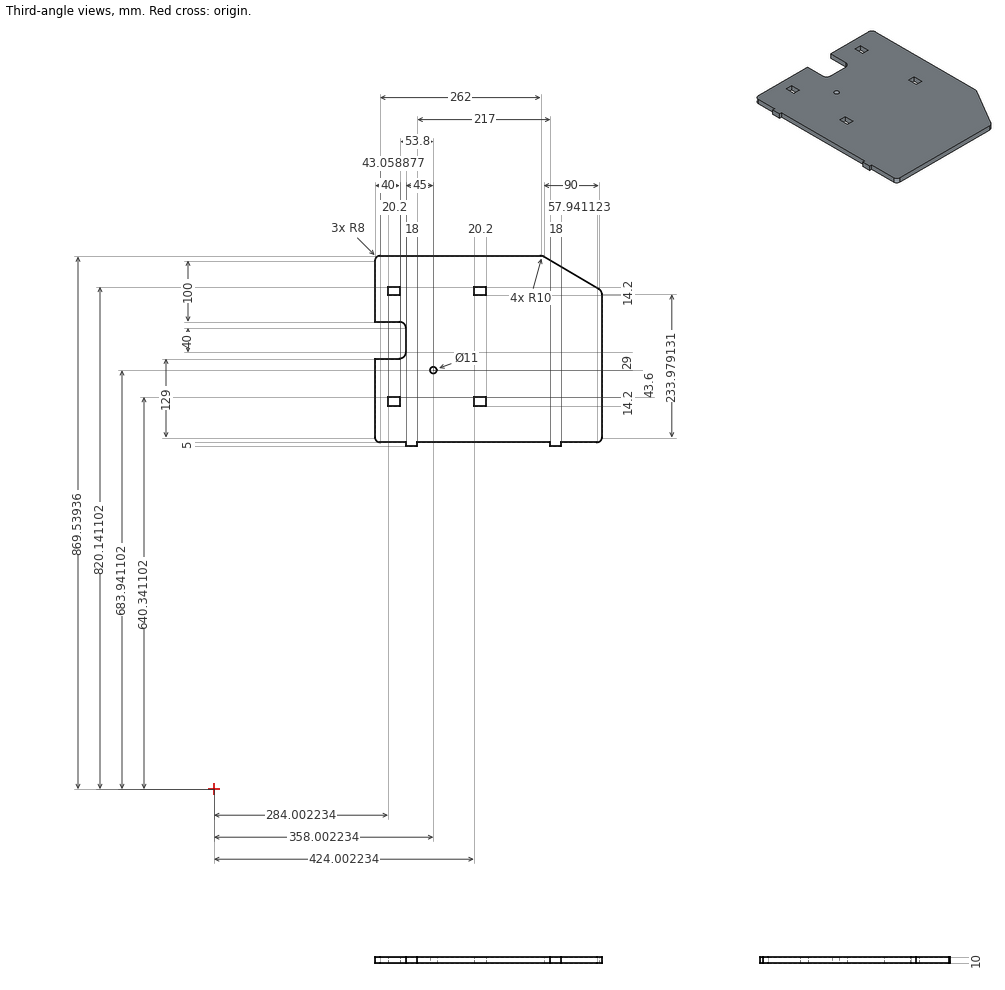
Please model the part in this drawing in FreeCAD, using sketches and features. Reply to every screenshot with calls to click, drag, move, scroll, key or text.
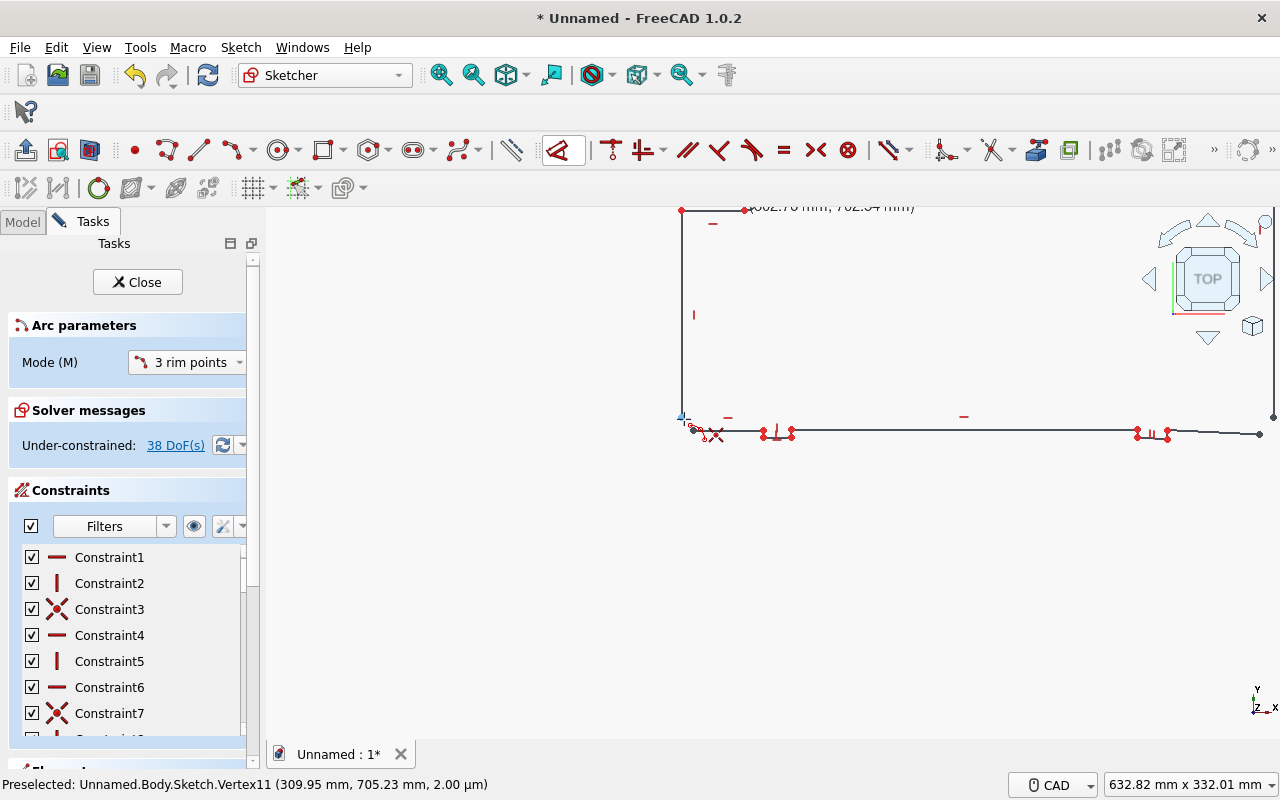
click(682, 417)
click(694, 431)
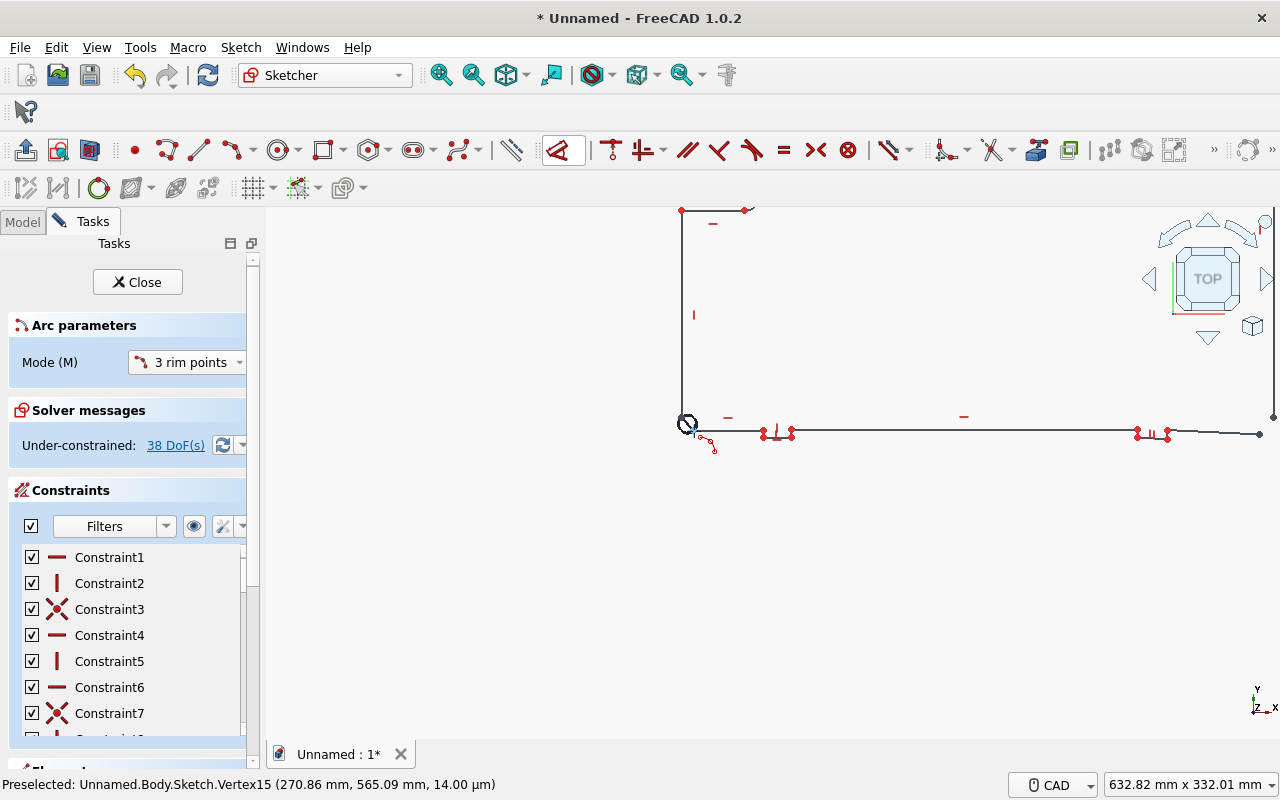
scroll(685, 426, up, 8)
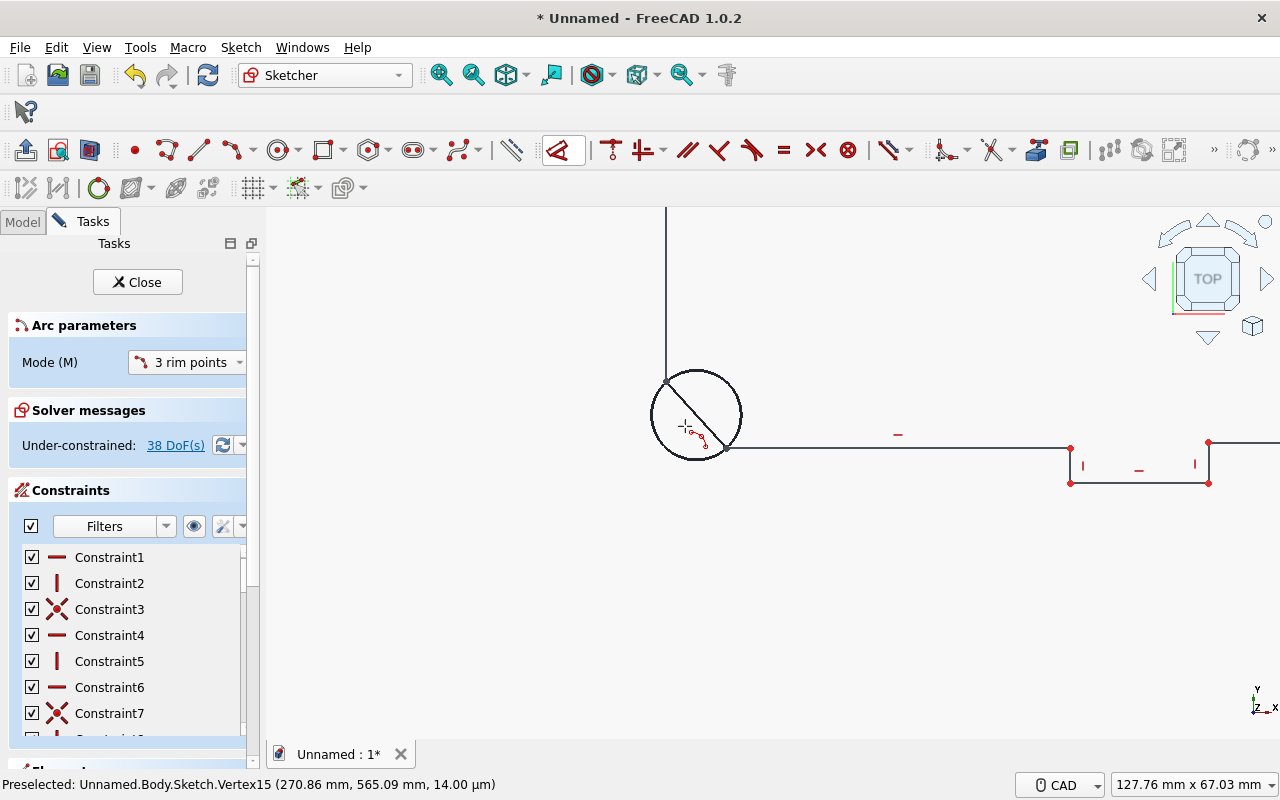
click(683, 423)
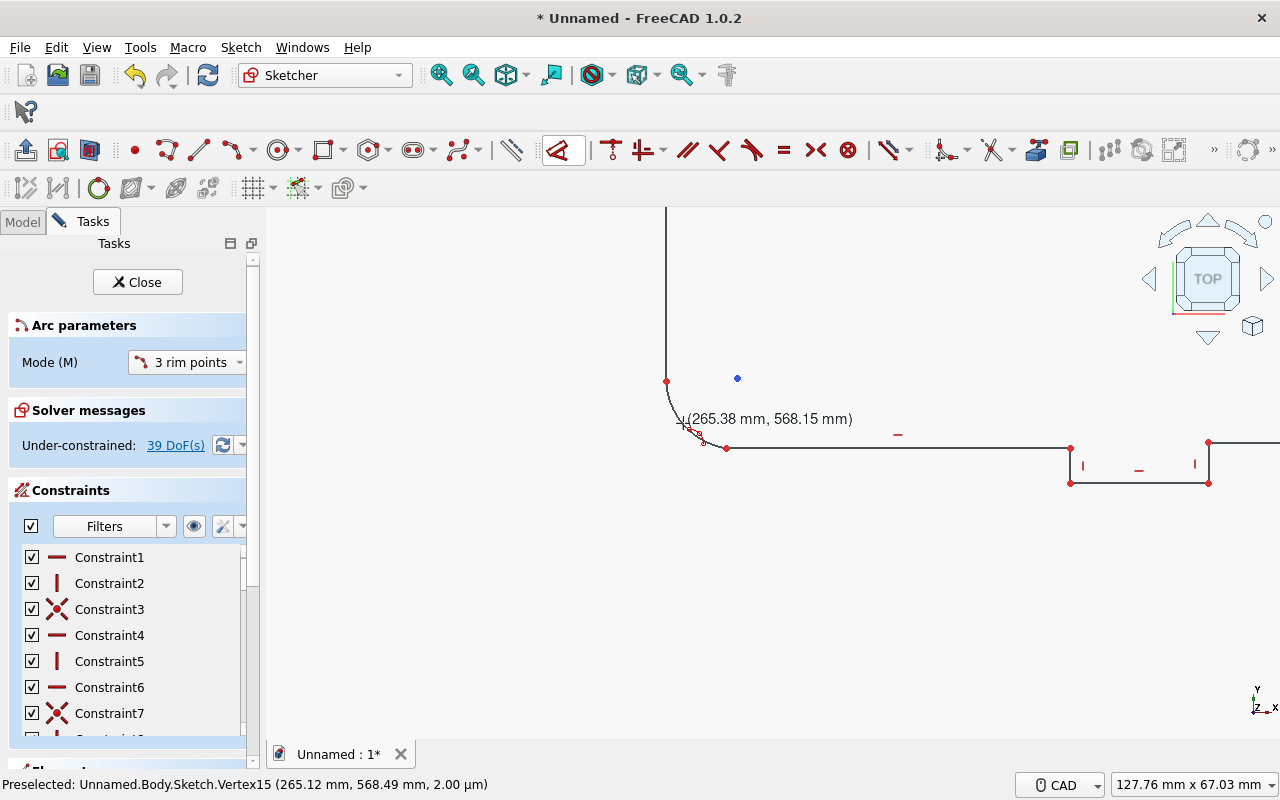
scroll(684, 420, down, 15)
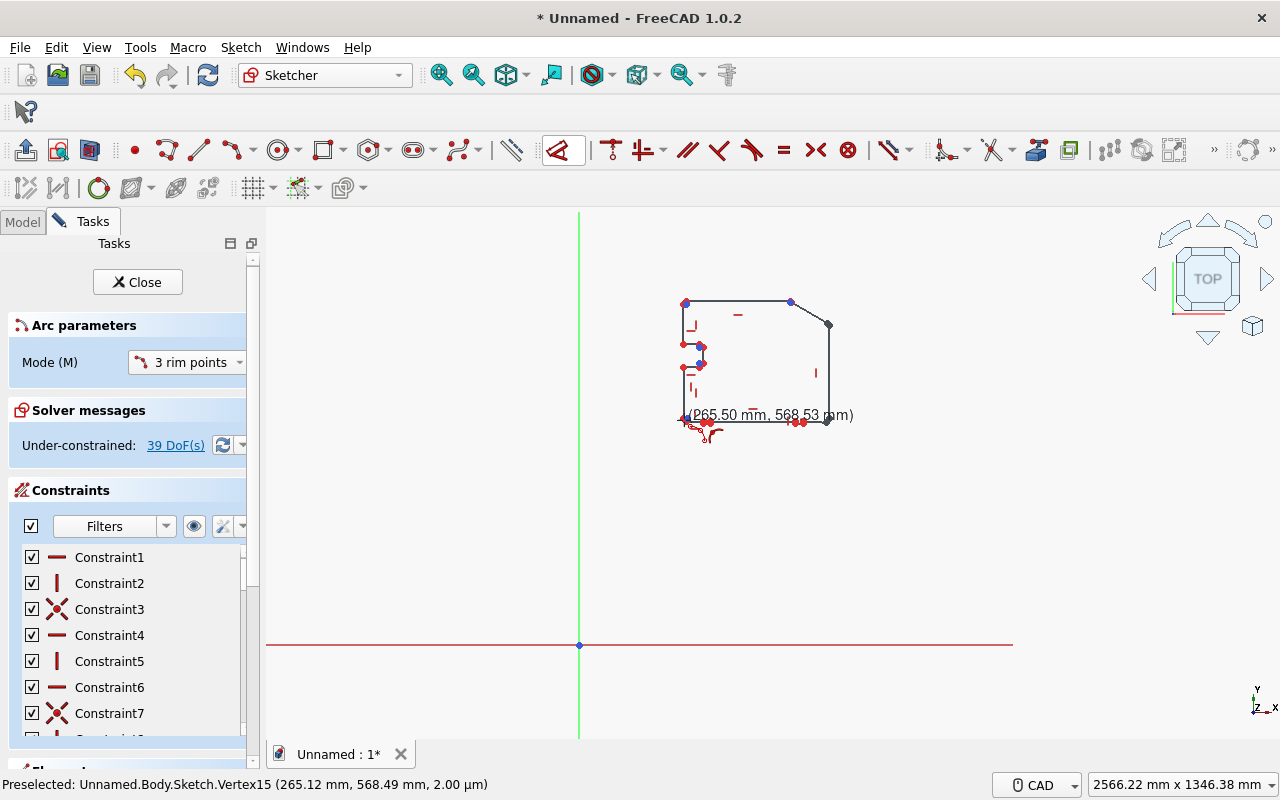
scroll(826, 421, up, 7)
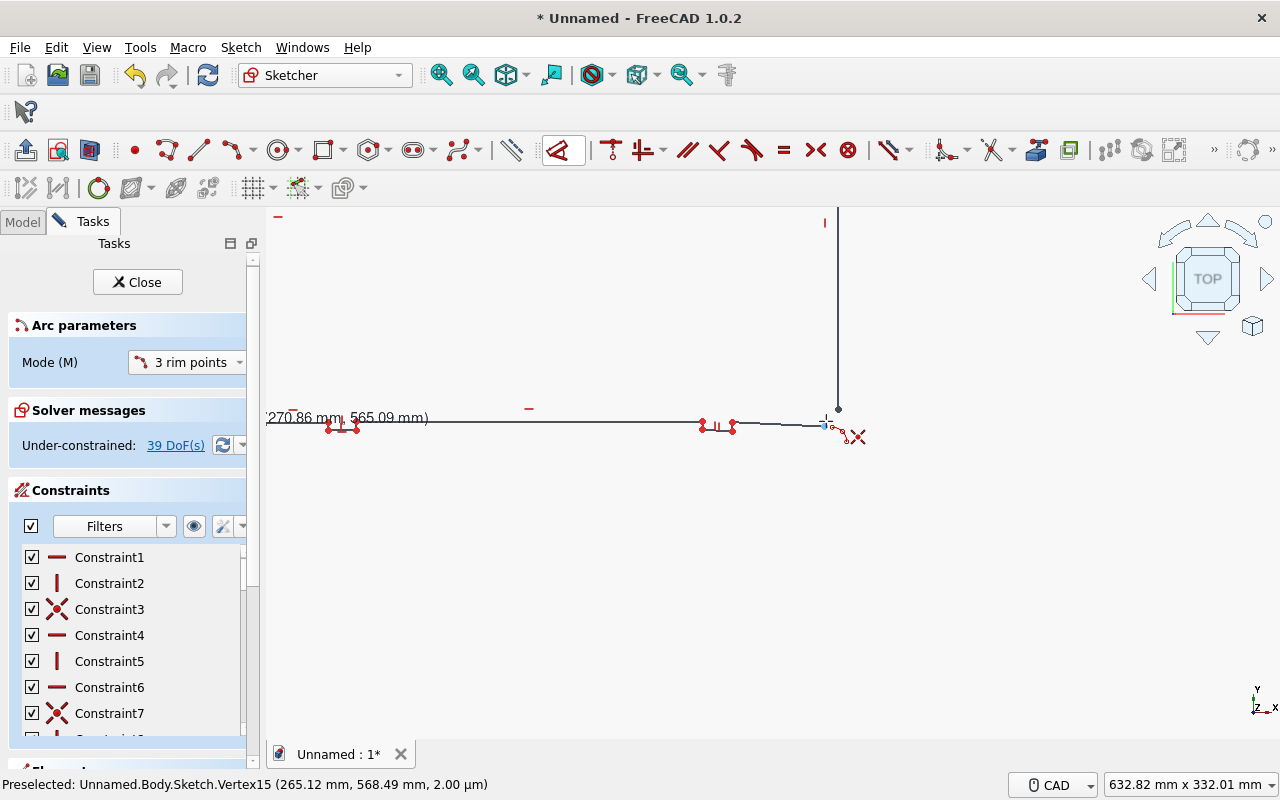
click(825, 427)
click(838, 410)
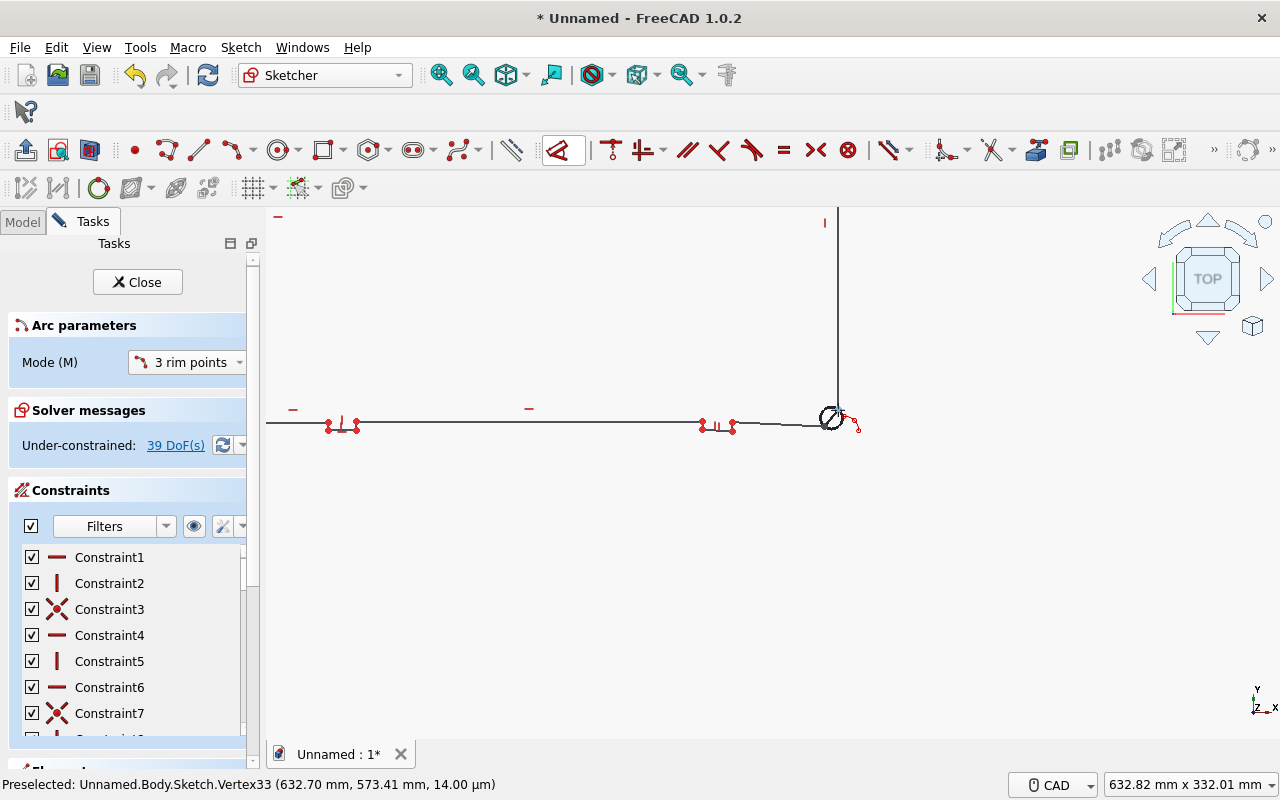
scroll(835, 418, up, 8)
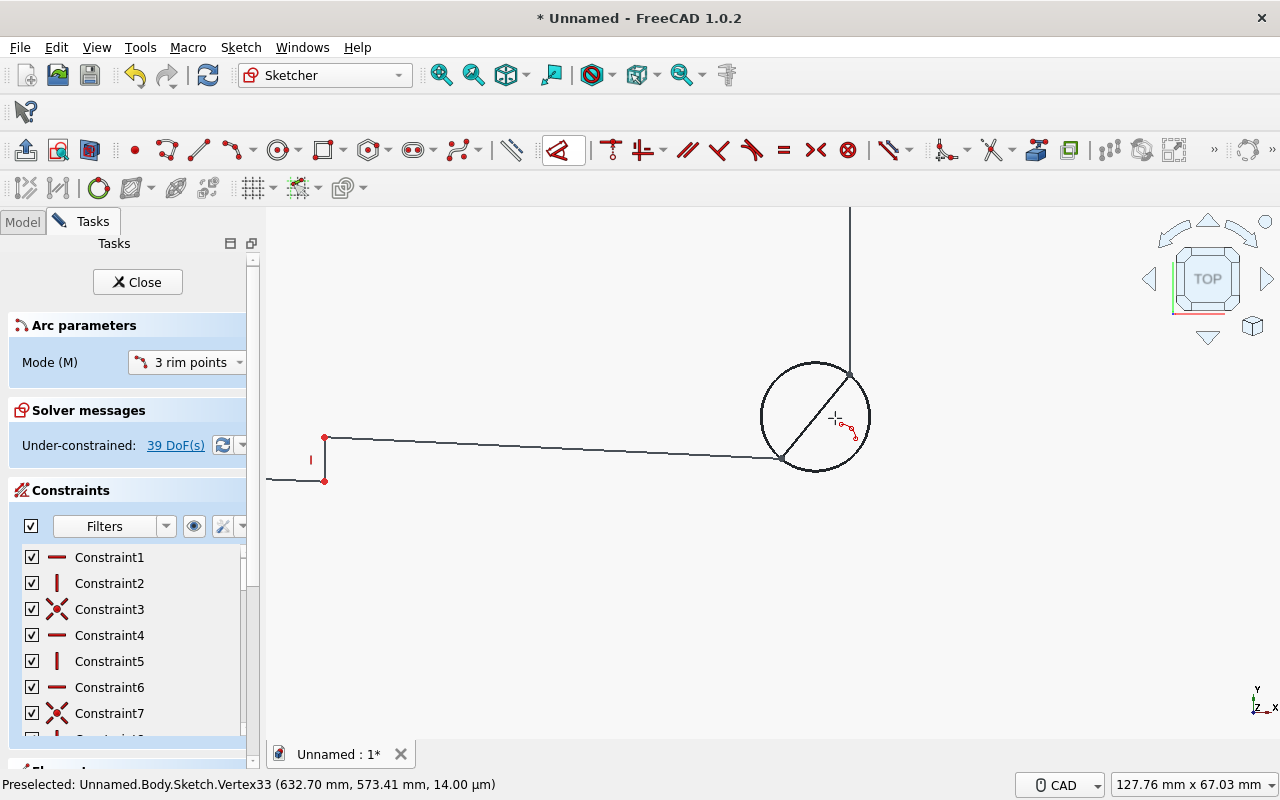
click(834, 416)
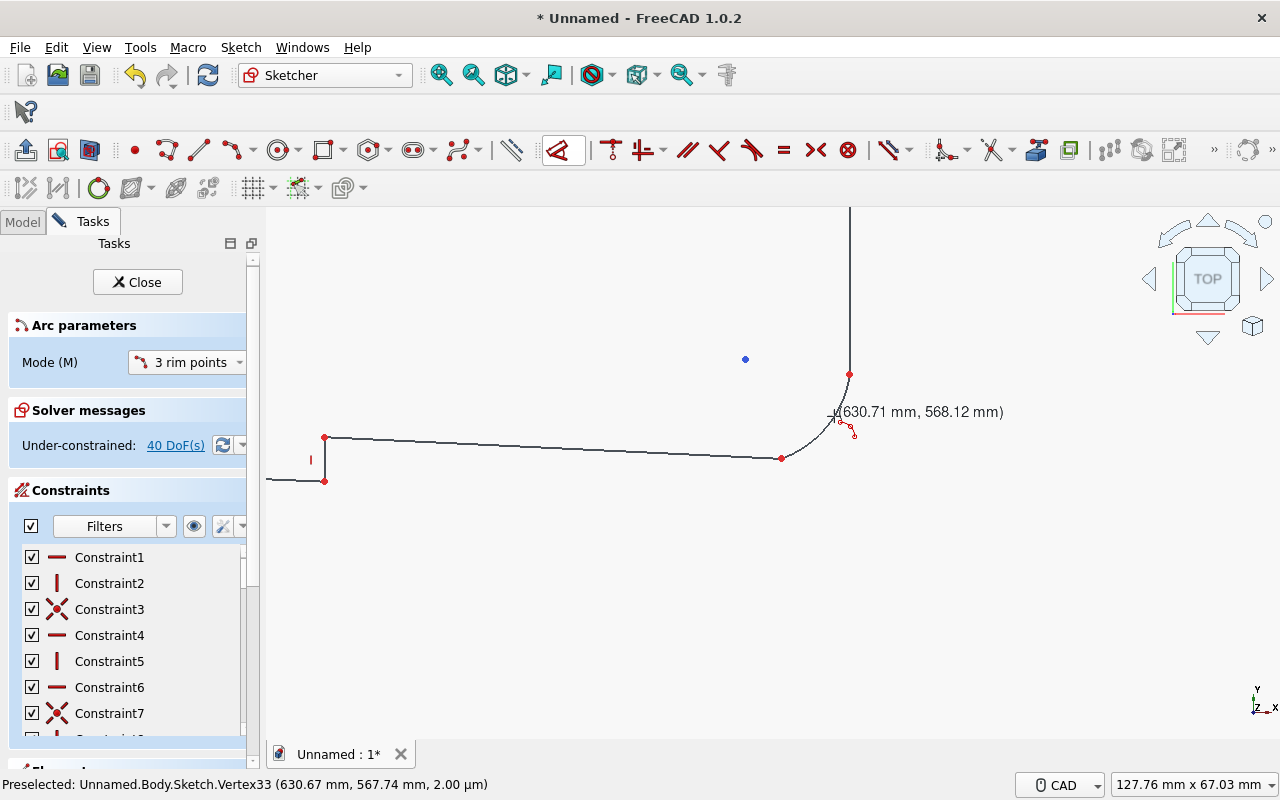
scroll(828, 421, down, 15)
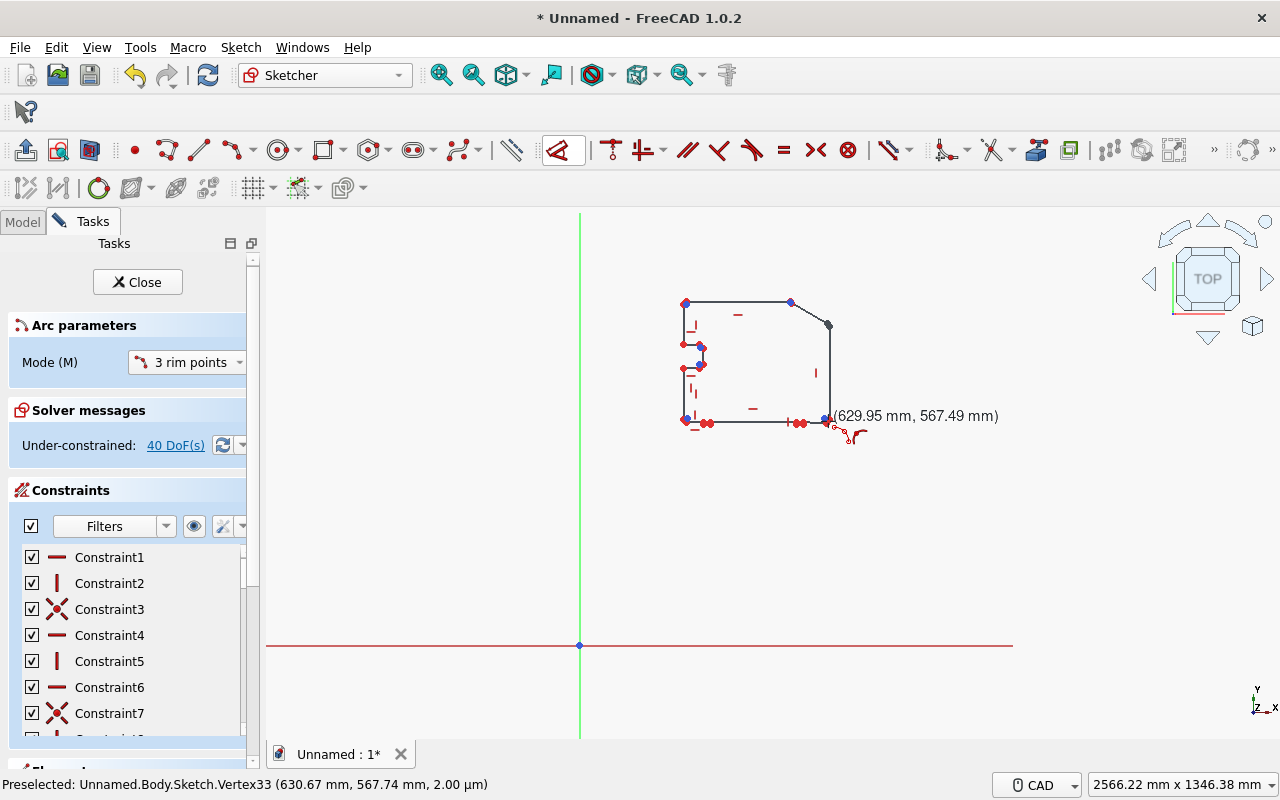
scroll(830, 326, up, 8)